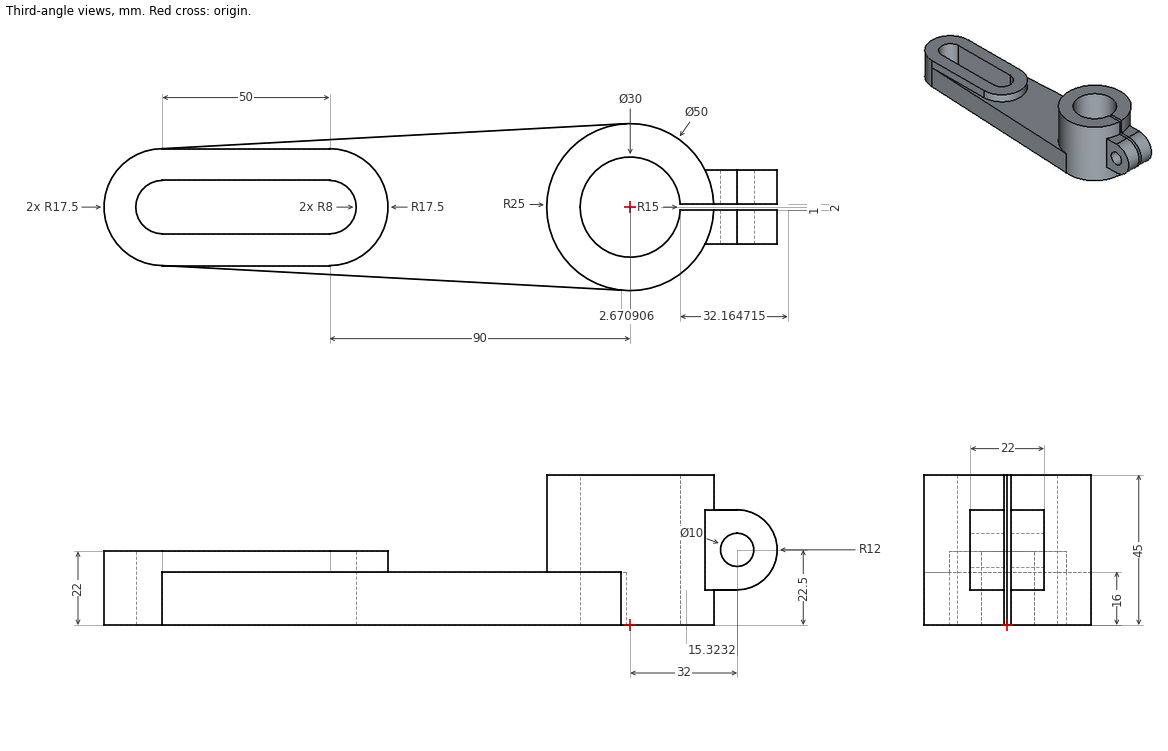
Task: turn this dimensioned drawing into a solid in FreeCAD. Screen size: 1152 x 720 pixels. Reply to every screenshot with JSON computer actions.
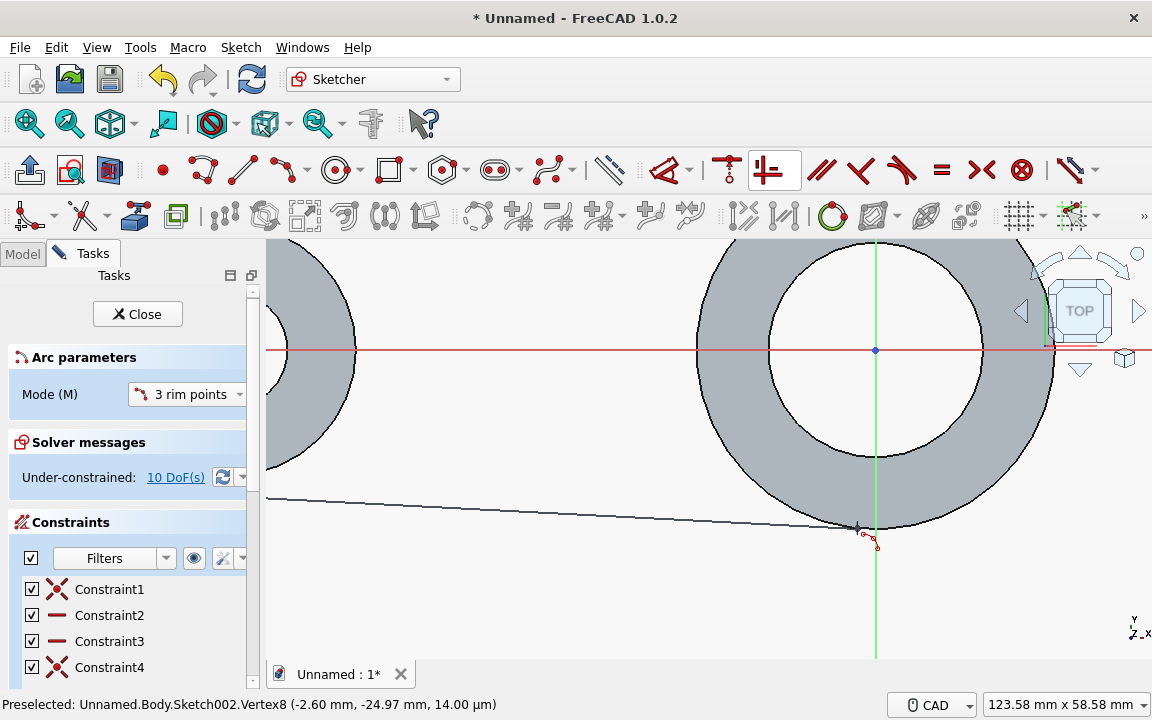
{"action": "scroll", "coordinate": [858, 530], "scroll_direction": "down", "scroll_amount": 4}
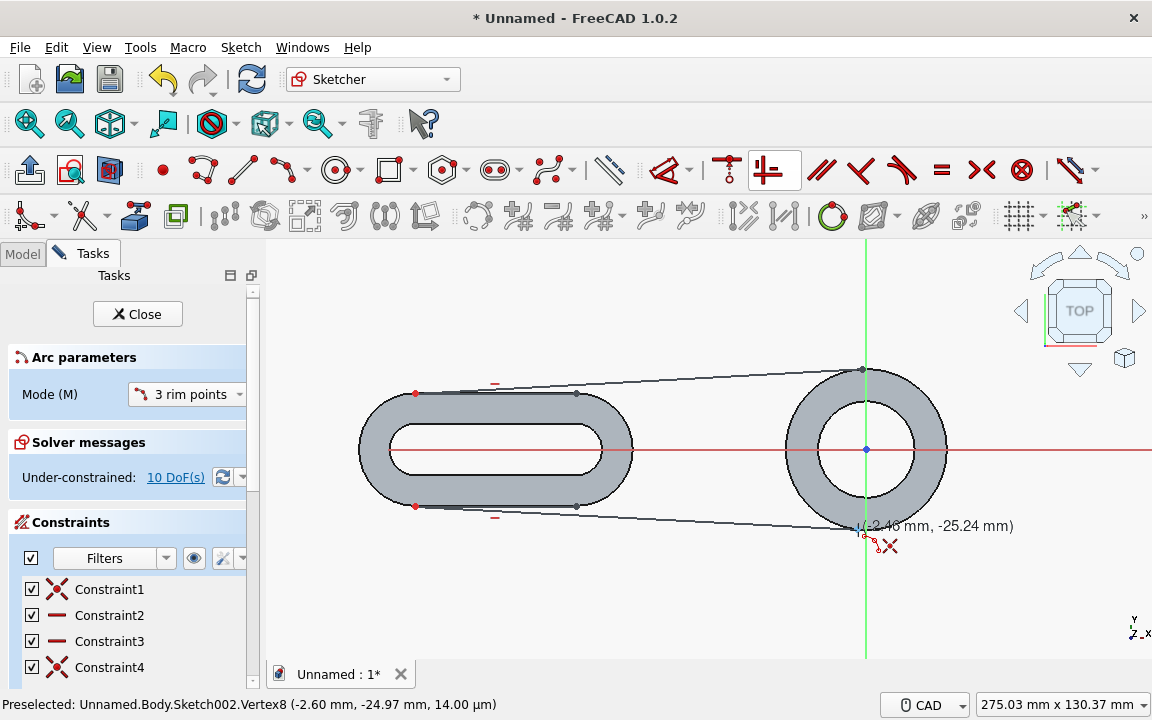
{"action": "scroll", "coordinate": [576, 393], "scroll_direction": "up", "scroll_amount": 4}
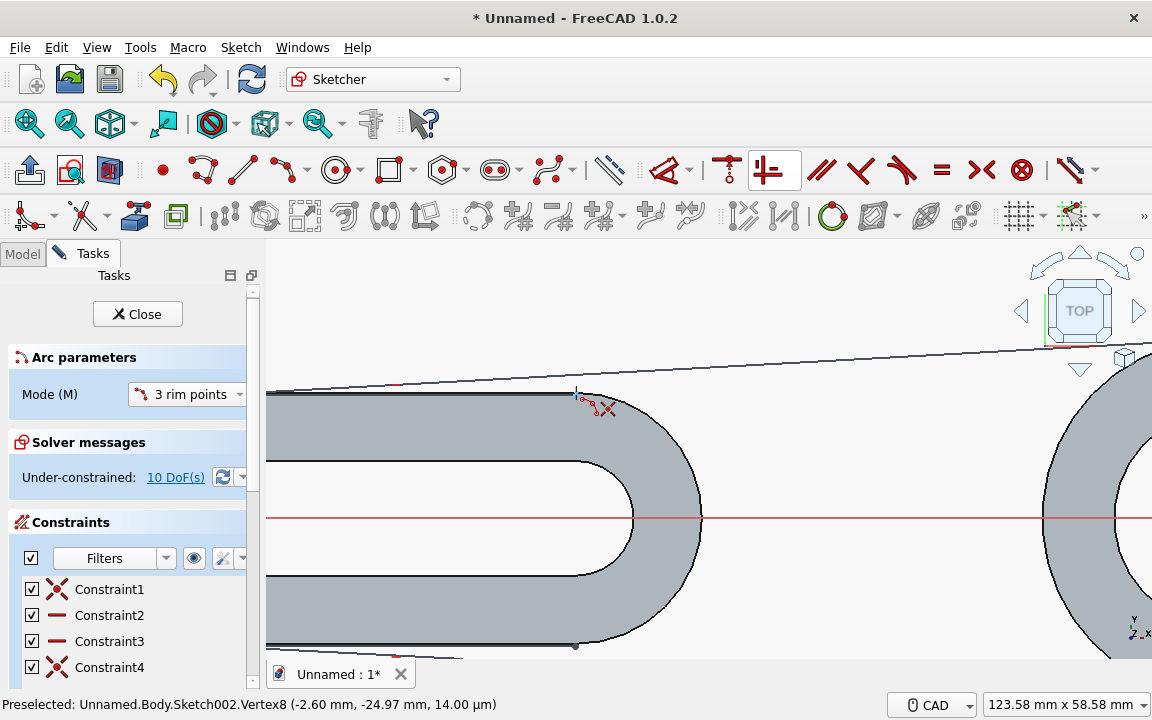
{"action": "left_click", "coordinate": [576, 395]}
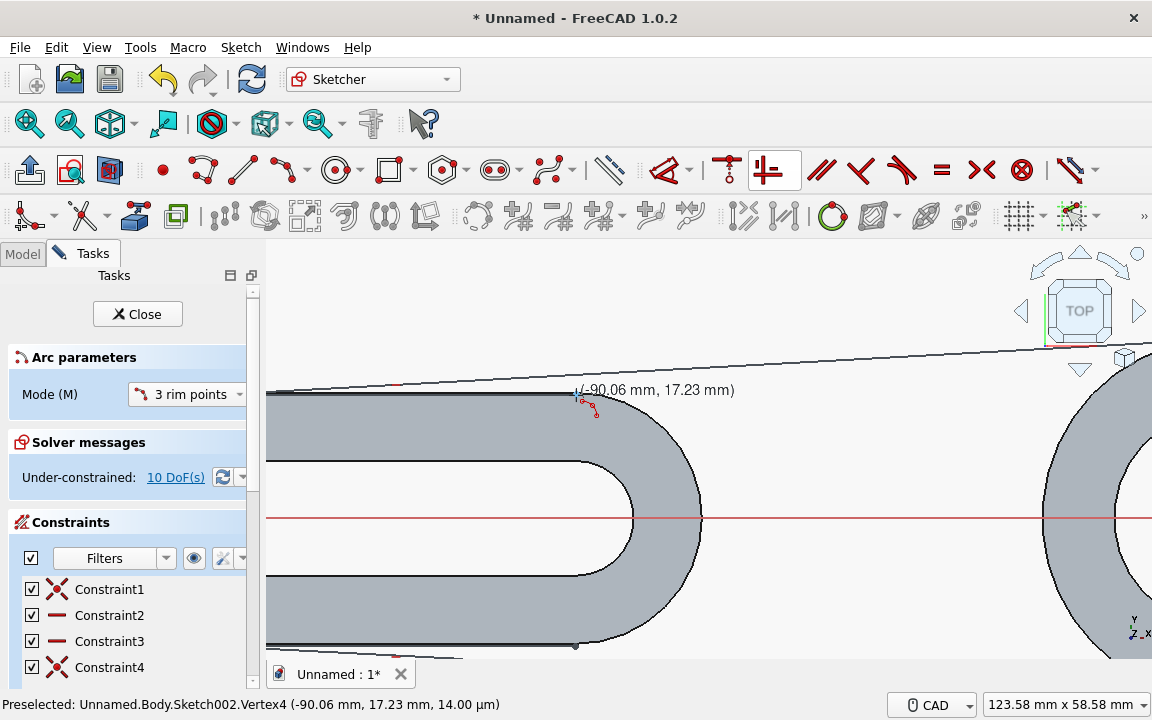
{"action": "scroll", "coordinate": [576, 393], "scroll_direction": "down", "scroll_amount": 4}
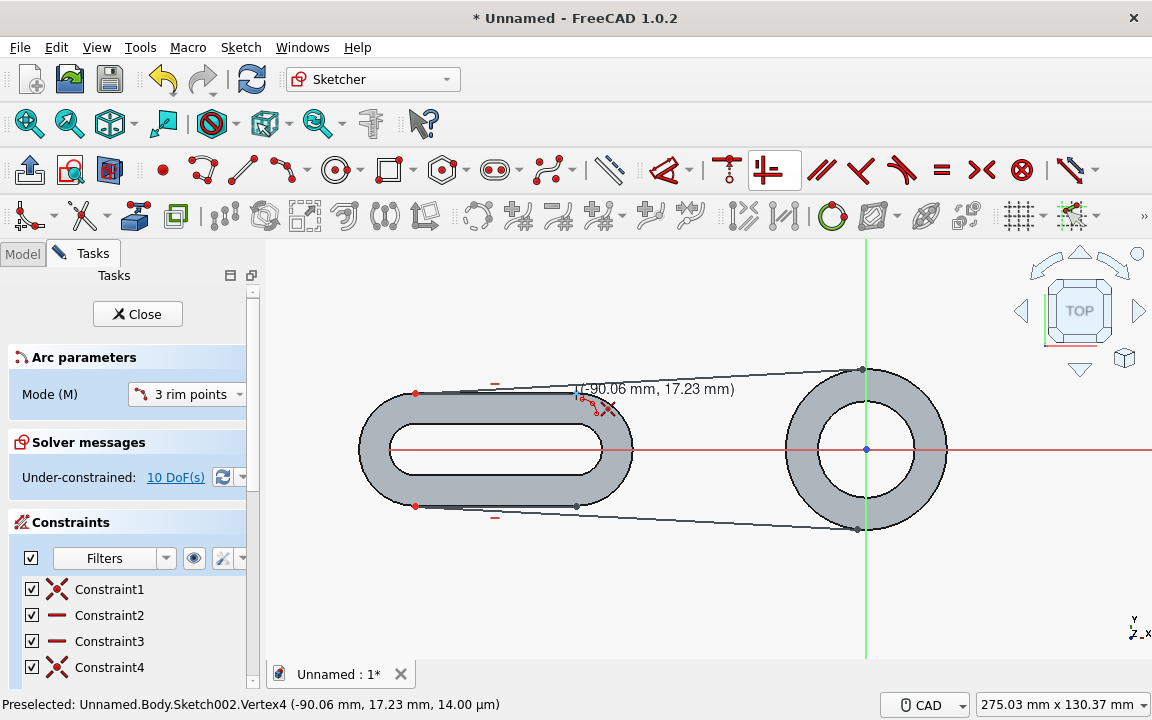
{"action": "scroll", "coordinate": [576, 506], "scroll_direction": "up", "scroll_amount": 4}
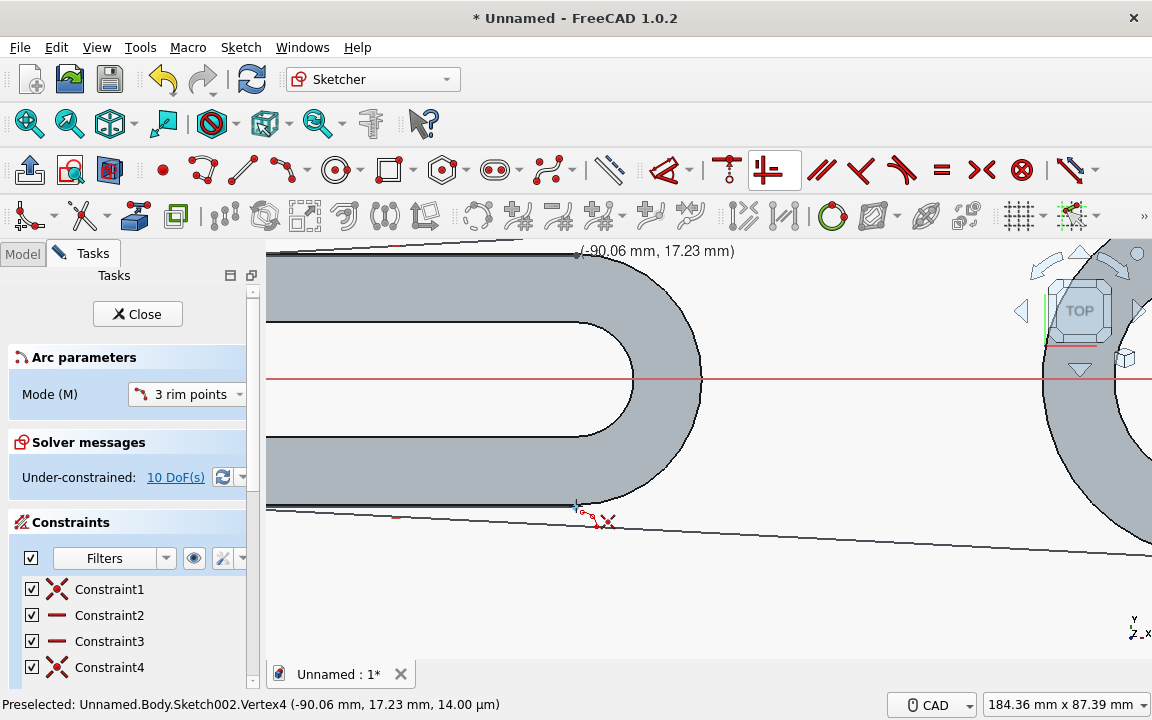
{"action": "left_click", "coordinate": [576, 507]}
{"action": "left_click", "coordinate": [696, 418]}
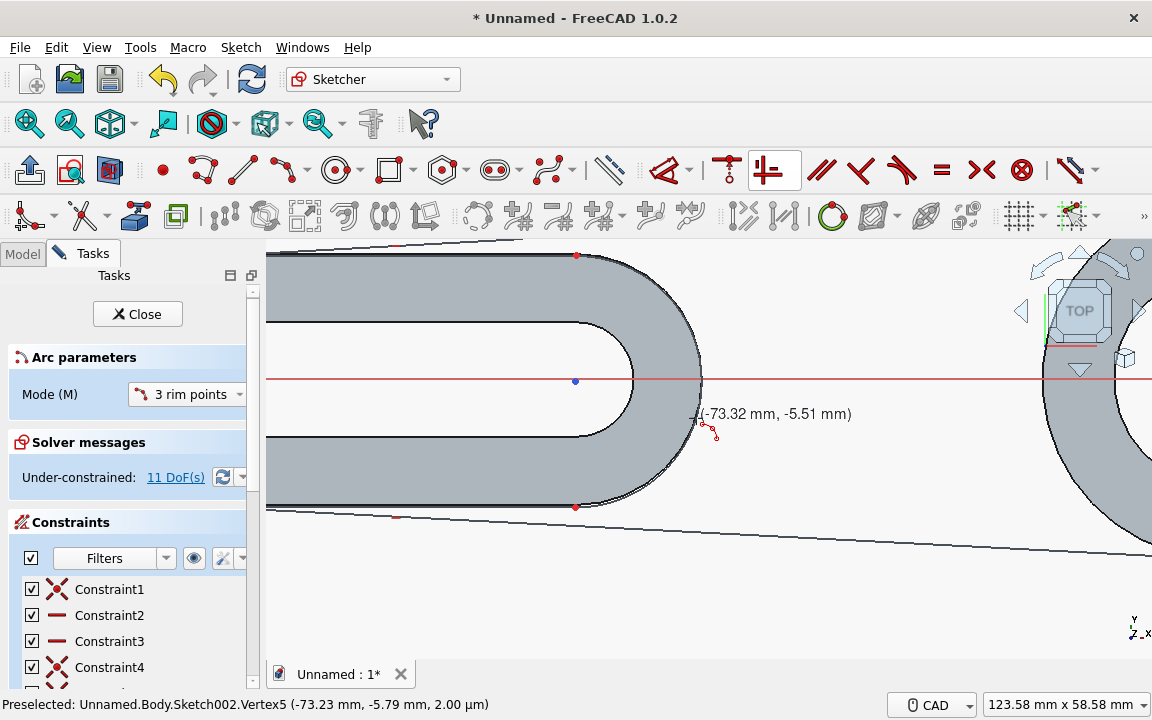
{"action": "scroll", "coordinate": [576, 506], "scroll_direction": "down", "scroll_amount": 4}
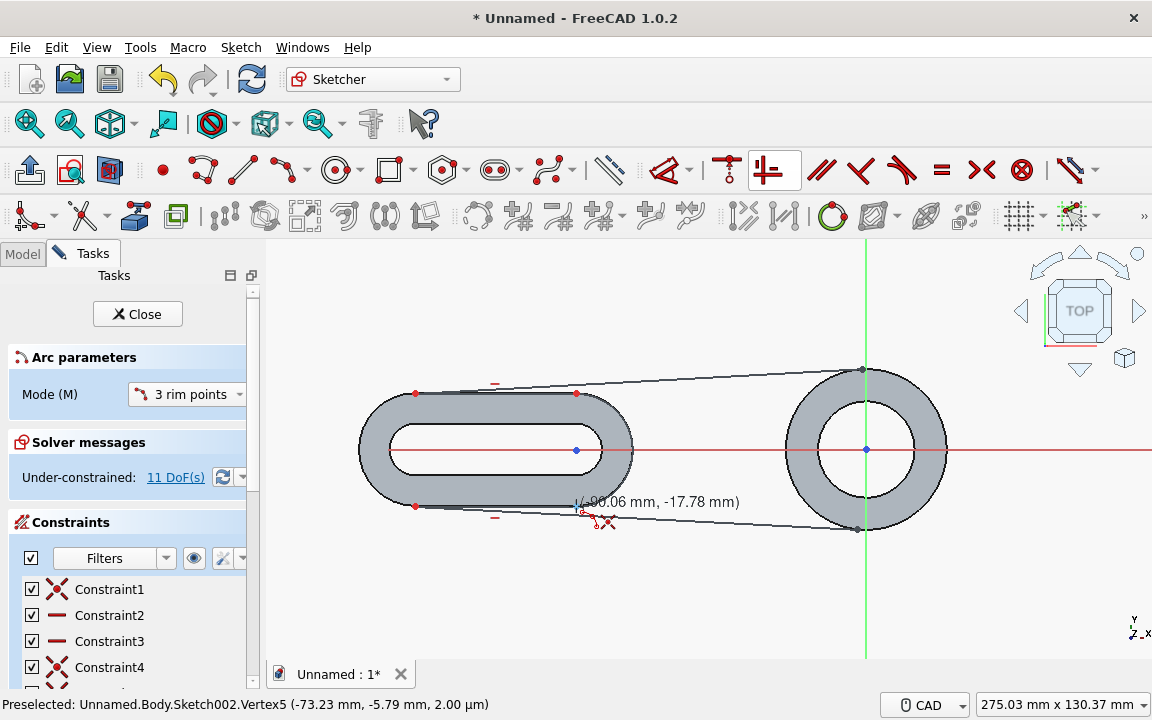
{"action": "scroll", "coordinate": [858, 530], "scroll_direction": "up", "scroll_amount": 4}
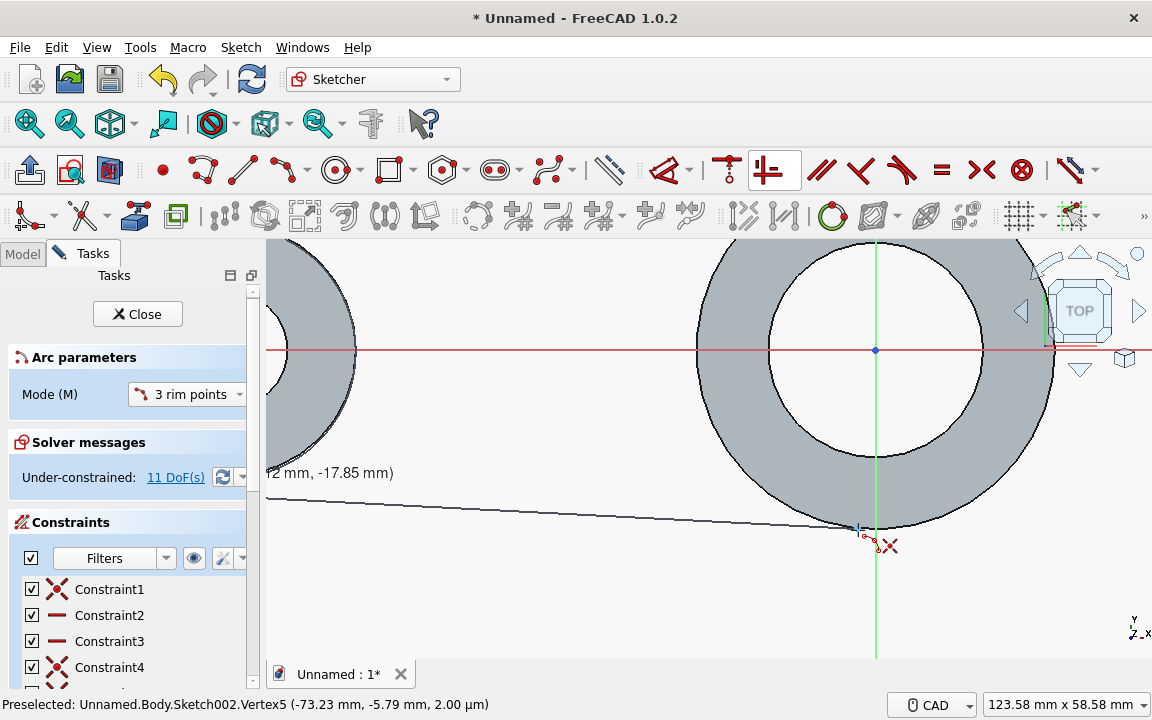
{"action": "left_click", "coordinate": [857, 529]}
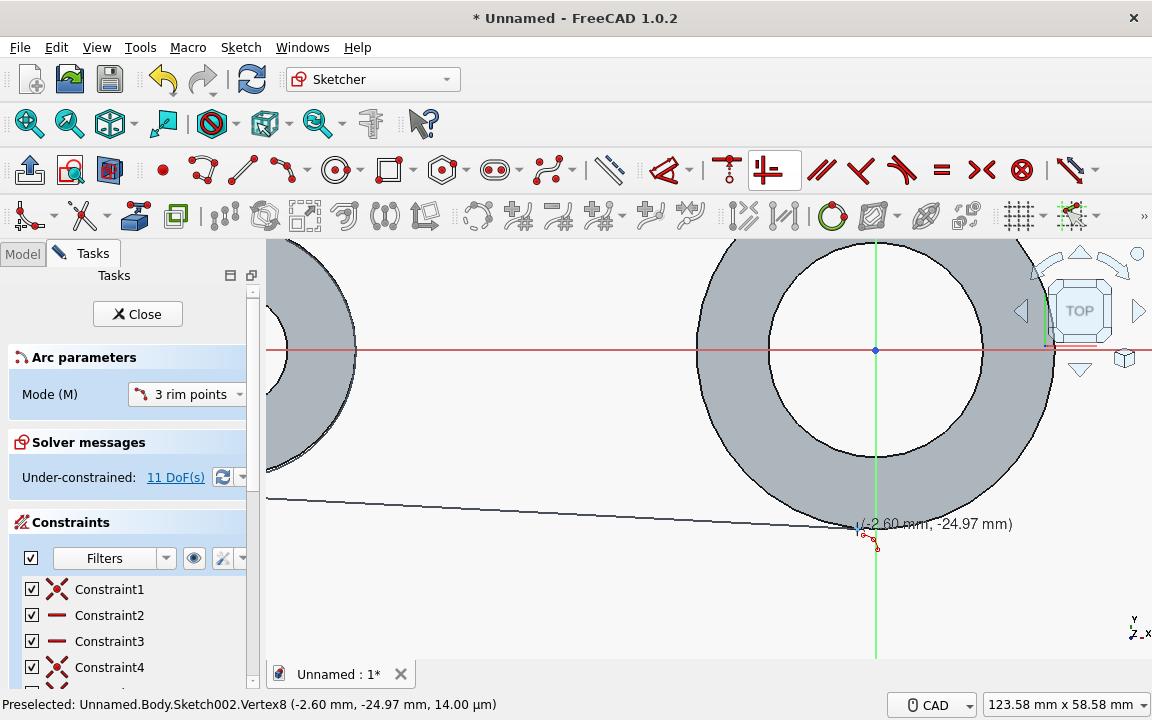
{"action": "scroll", "coordinate": [858, 530], "scroll_direction": "down", "scroll_amount": 4}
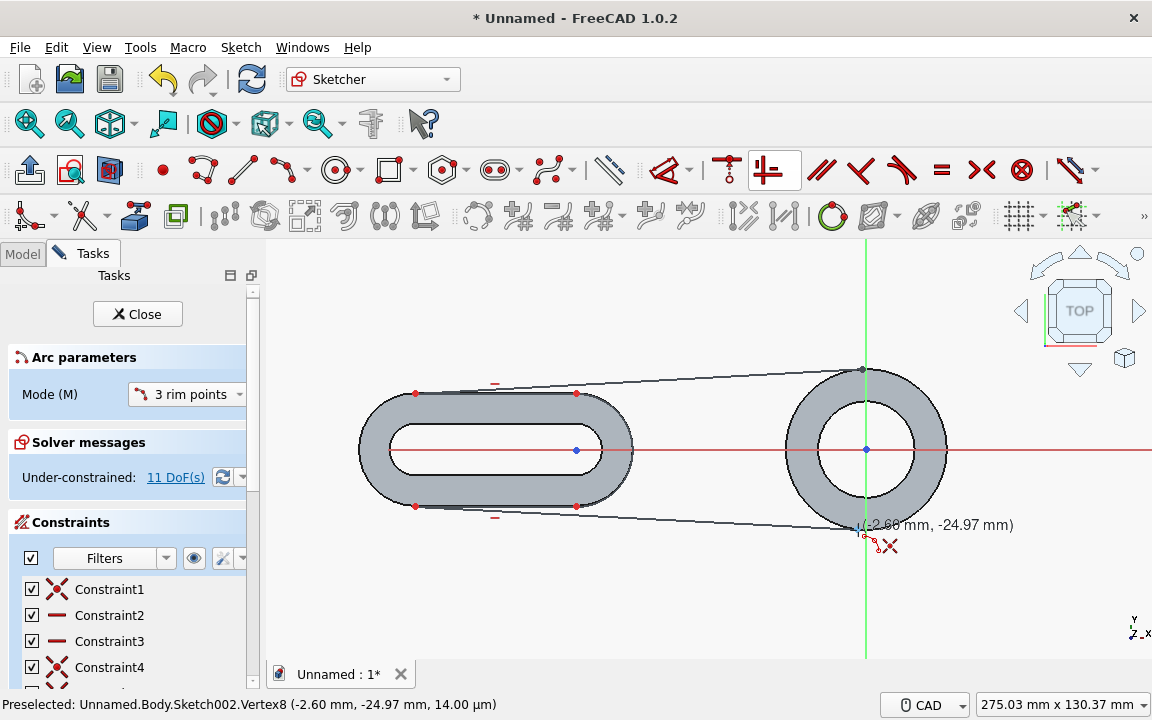
{"action": "scroll", "coordinate": [862, 369], "scroll_direction": "up", "scroll_amount": 7}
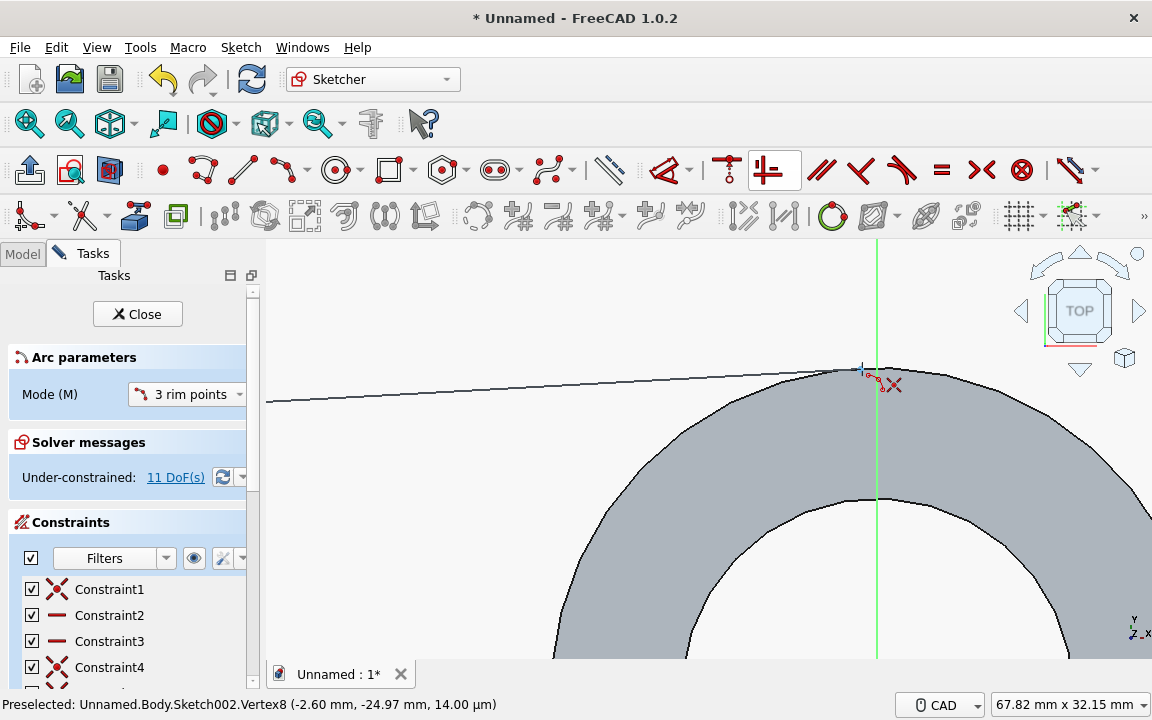
{"action": "left_click", "coordinate": [860, 369]}